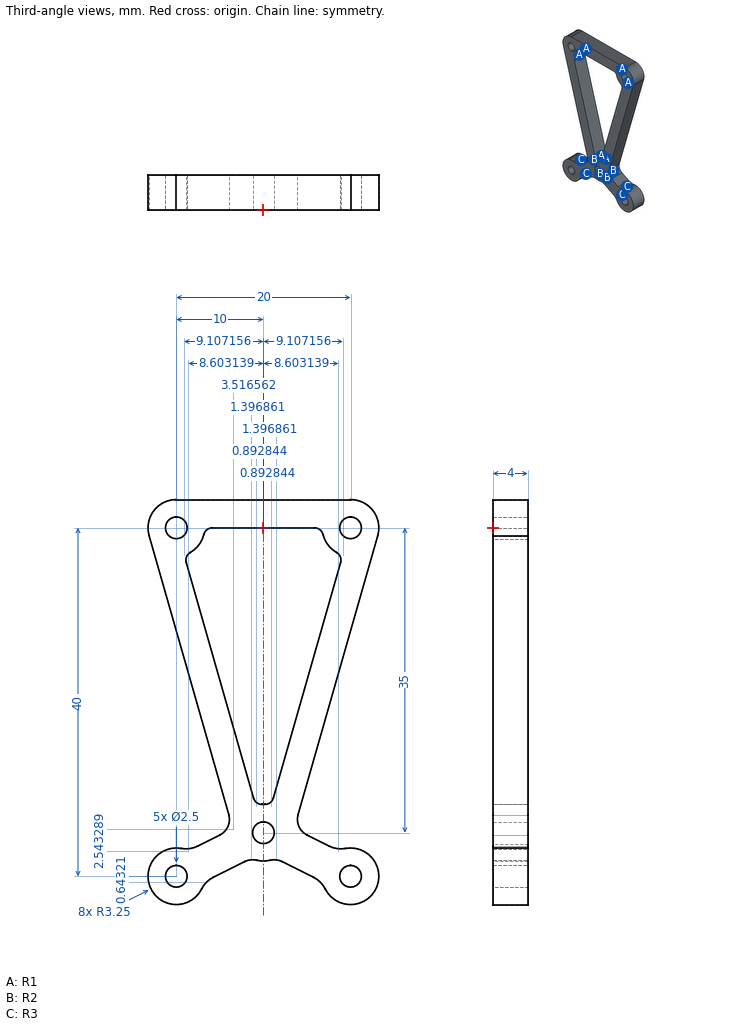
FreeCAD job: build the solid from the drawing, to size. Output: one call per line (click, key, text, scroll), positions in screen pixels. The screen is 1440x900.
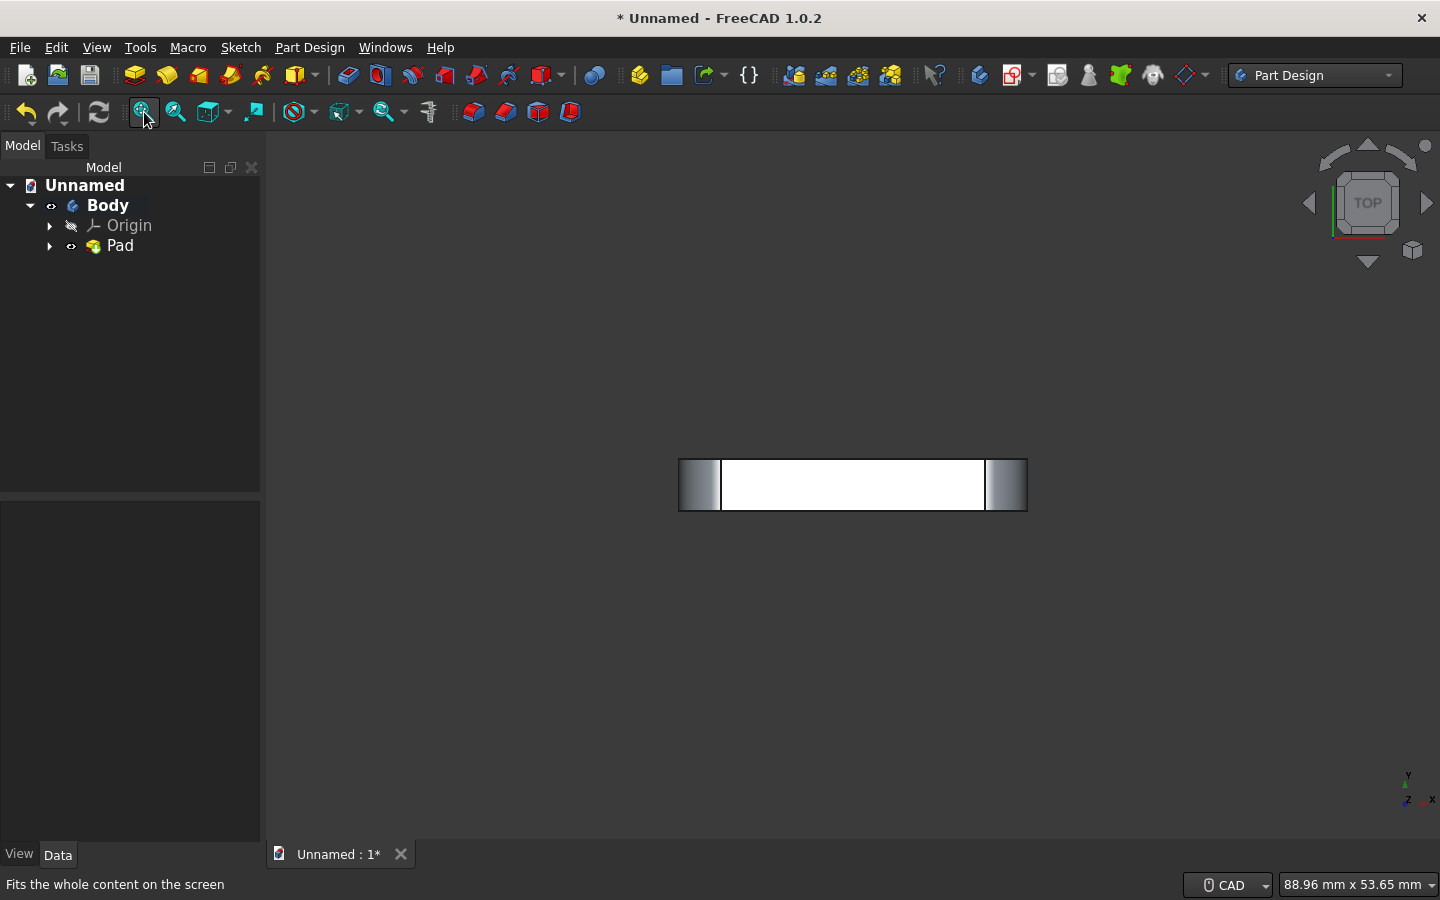
key(1)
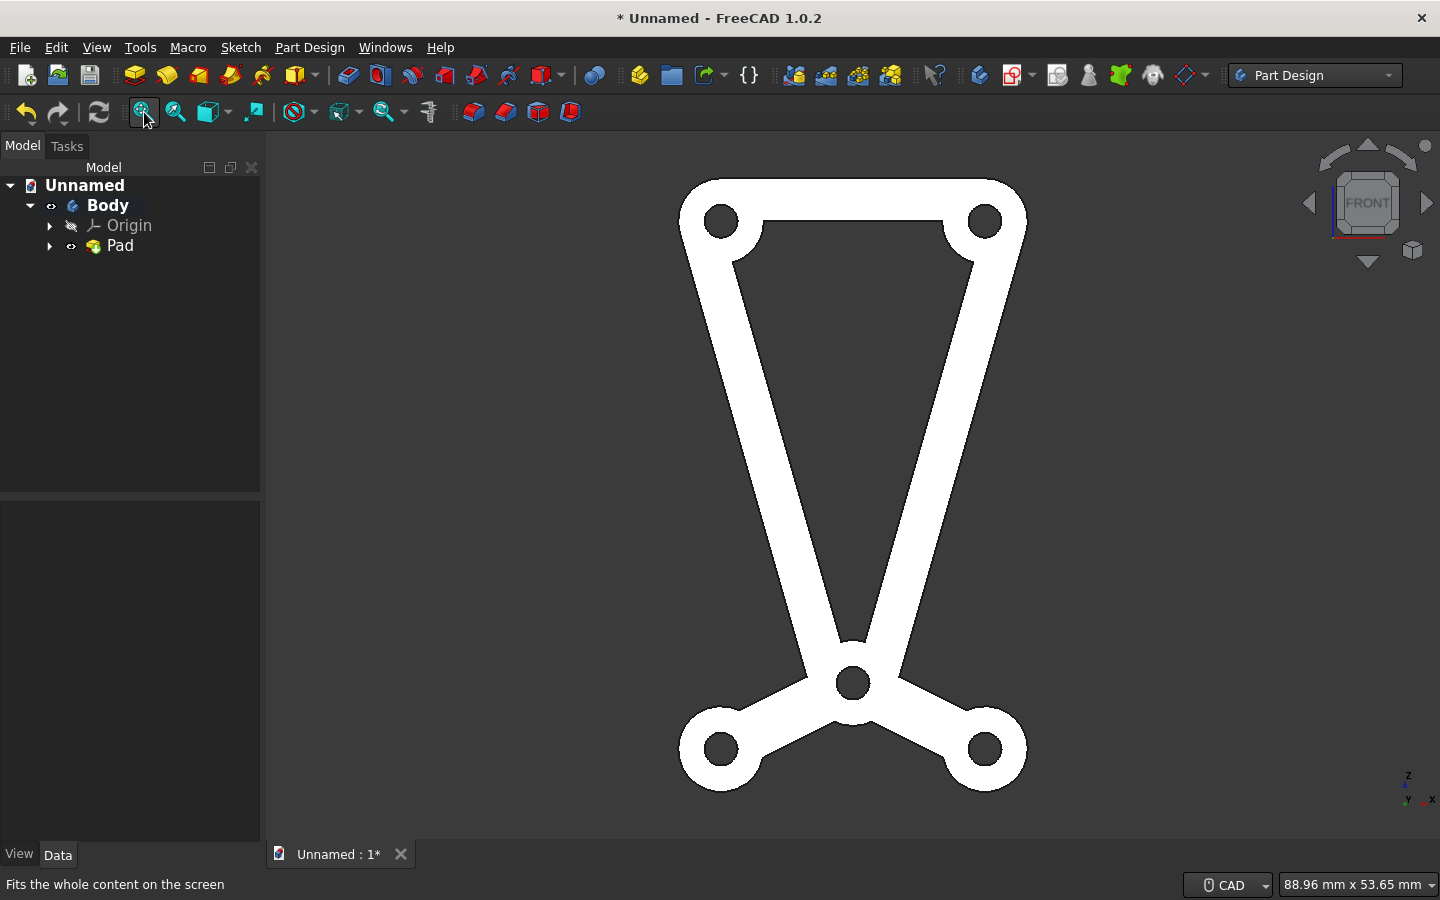
key(3)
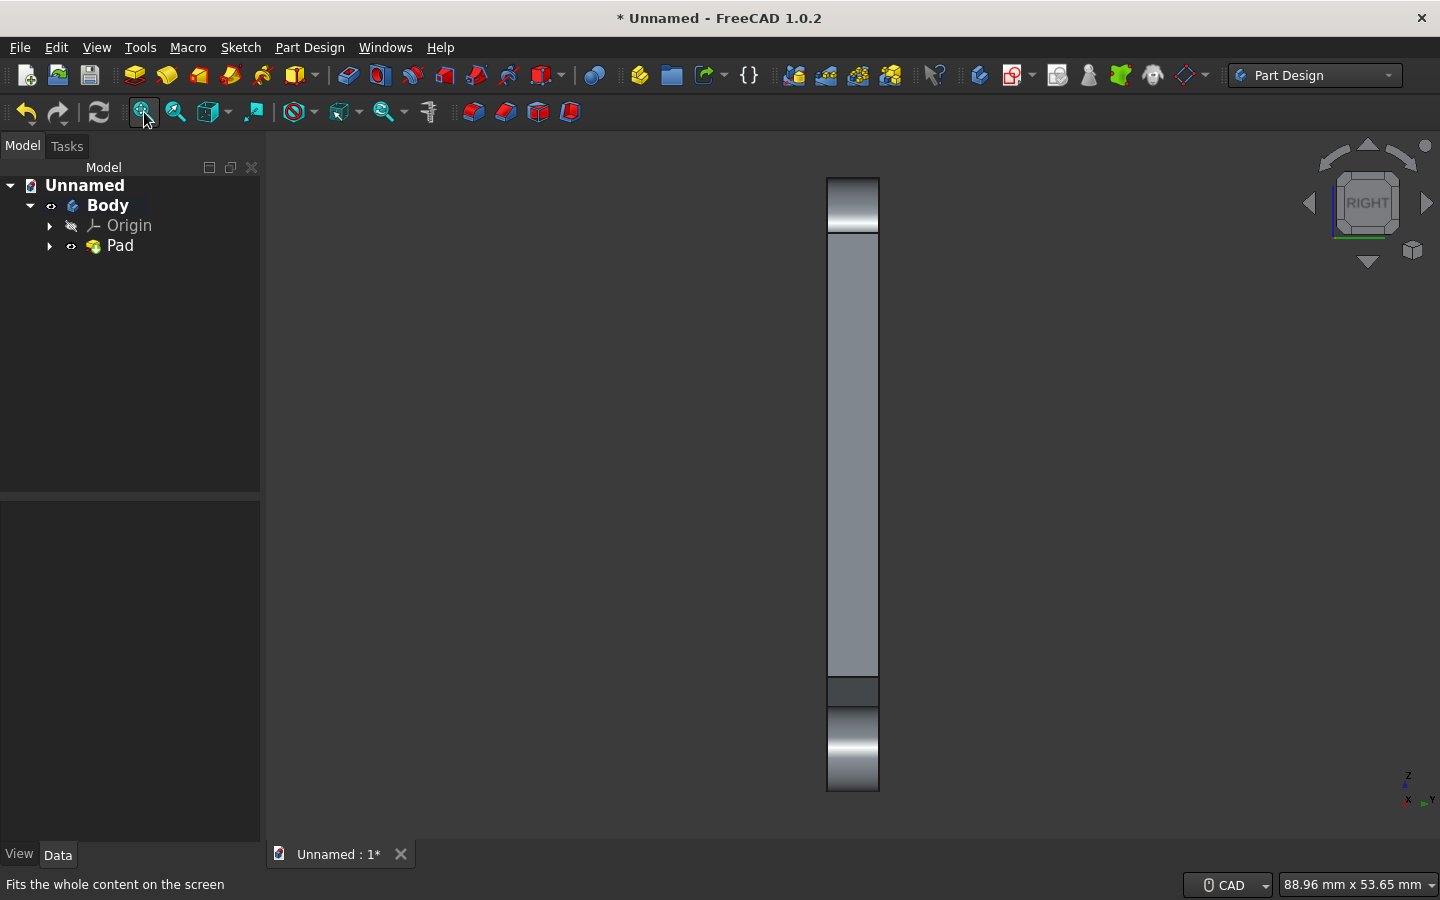
key(5)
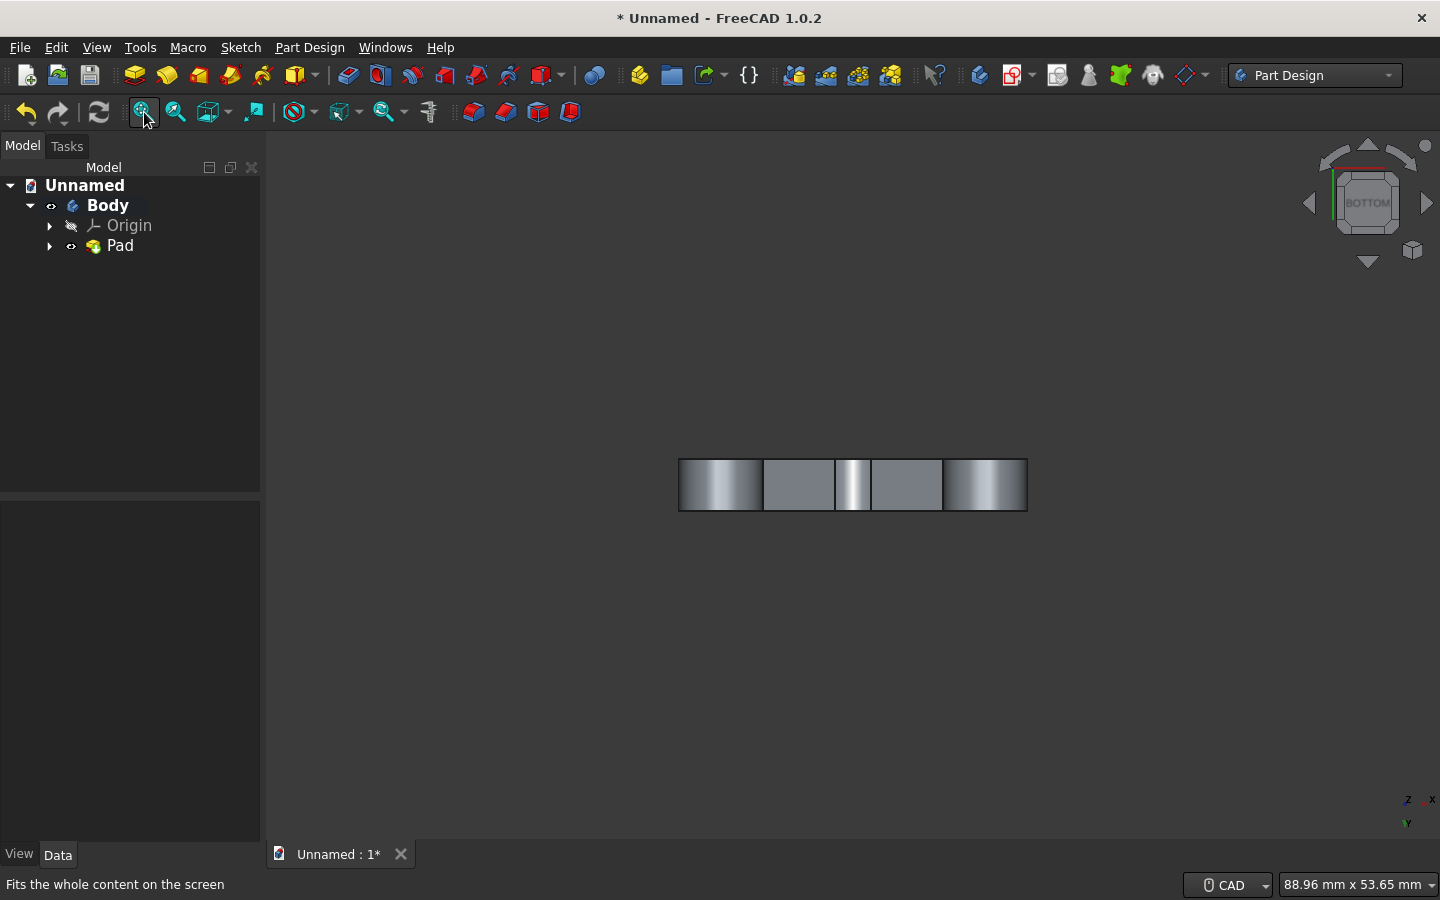
click(144, 112)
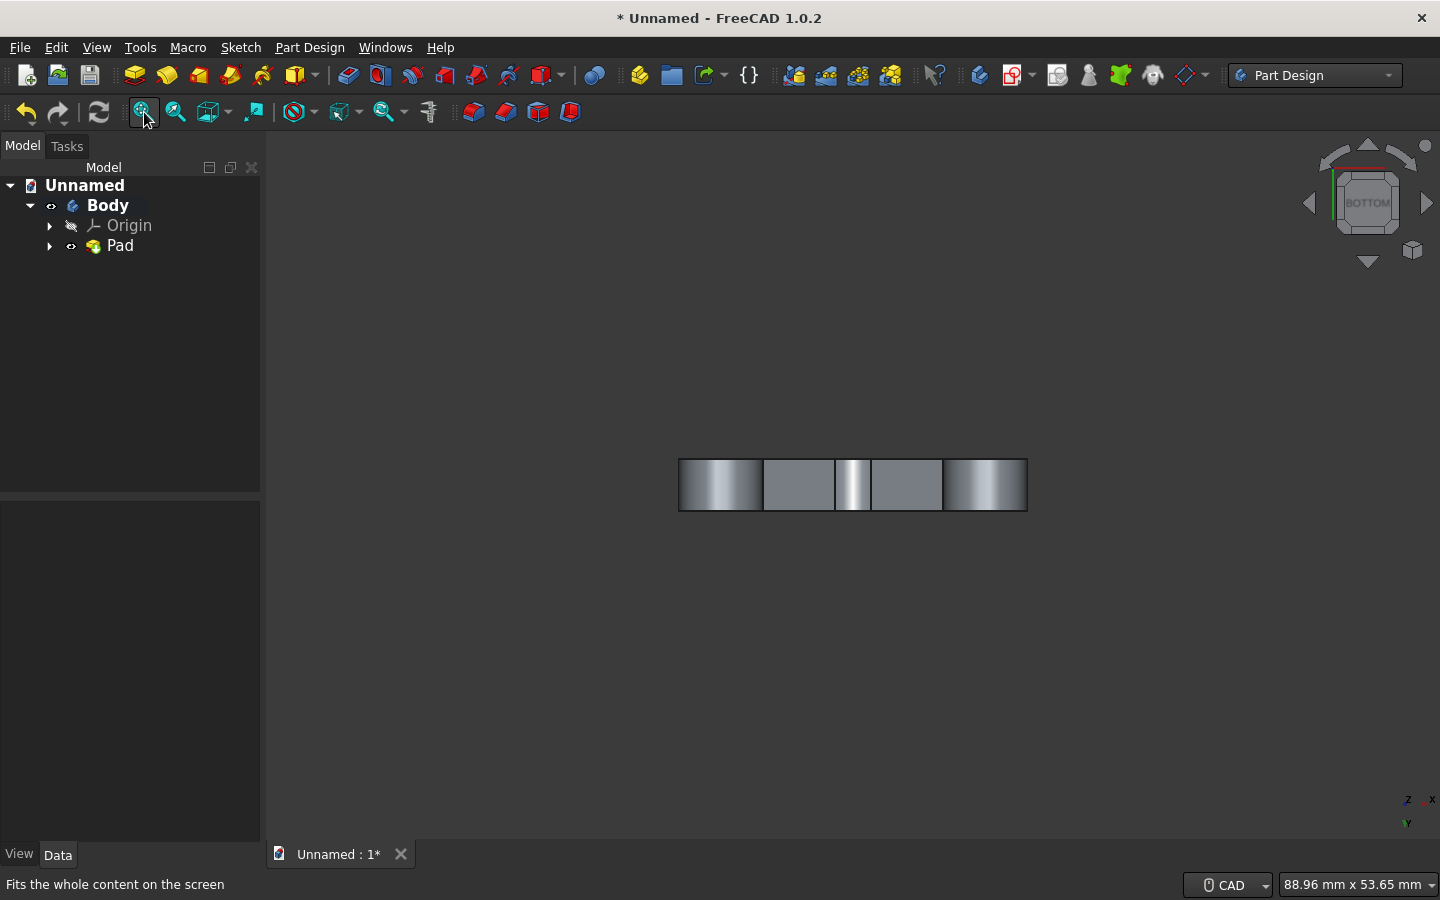
key(4)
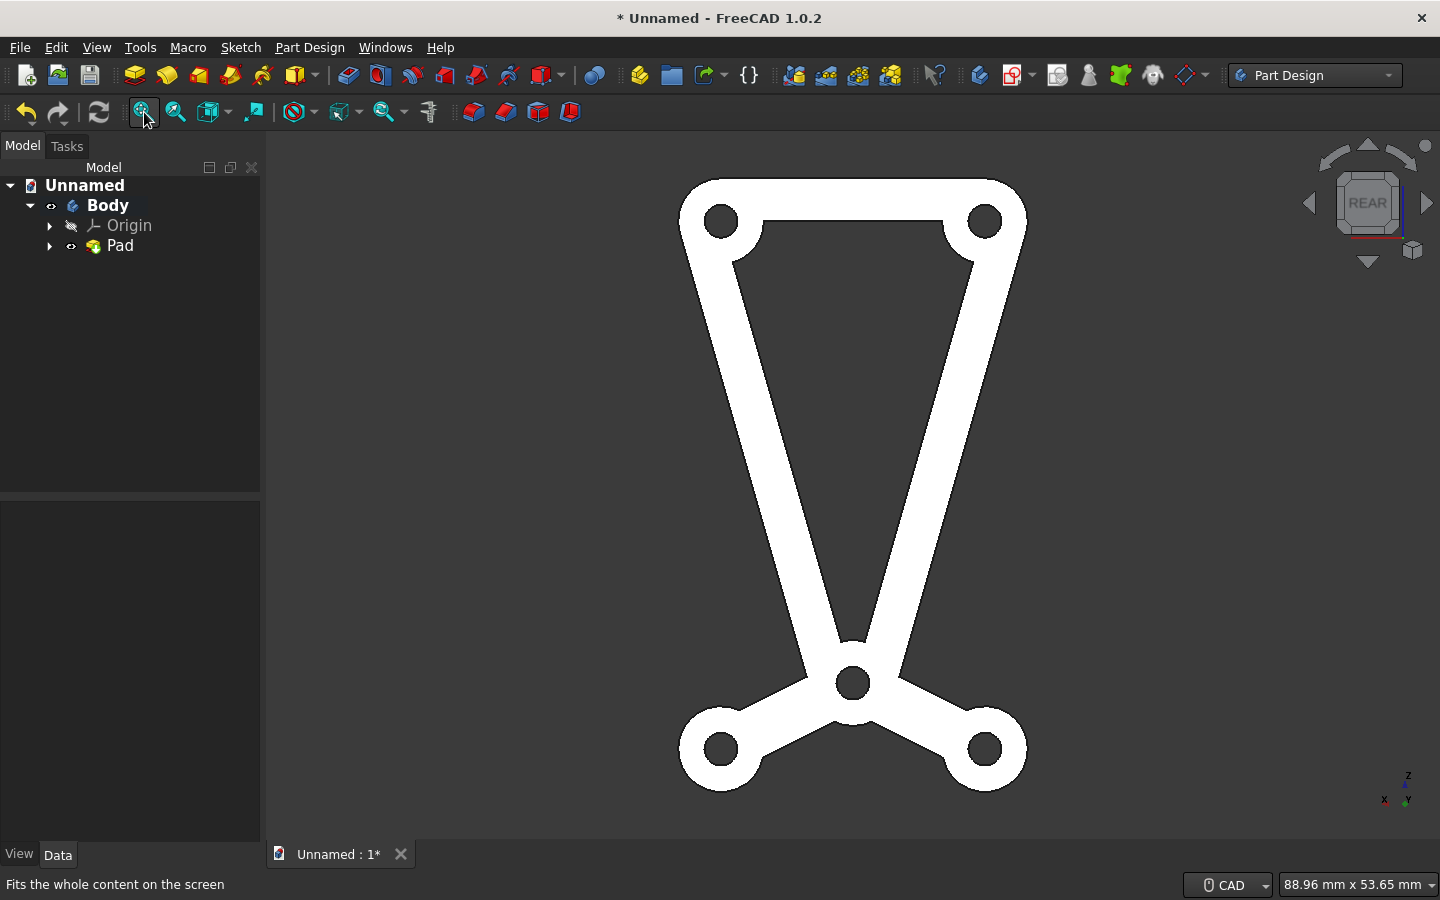
key(6)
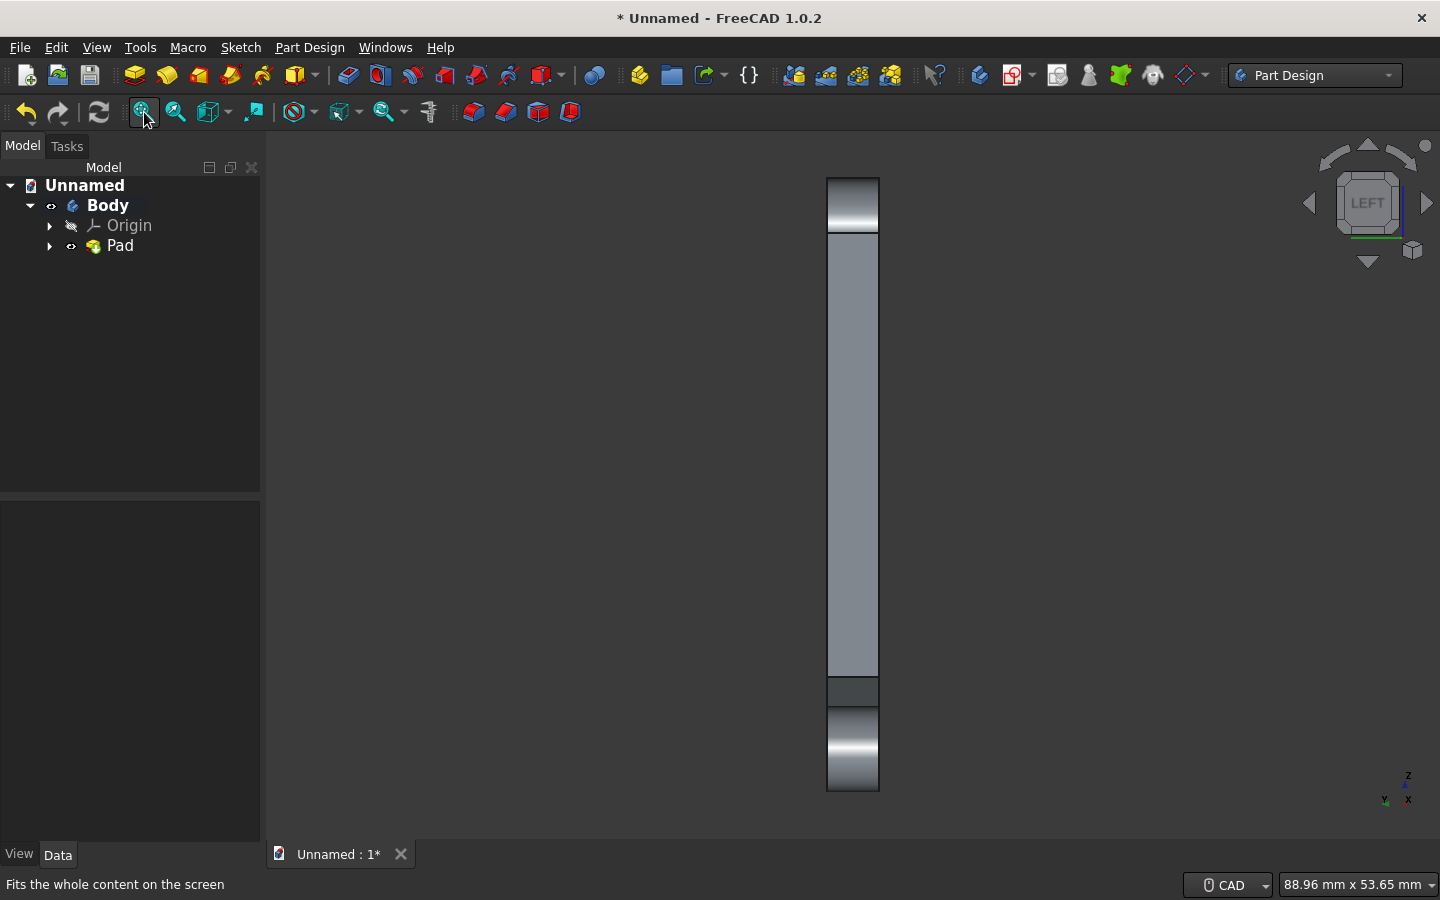
key(v)
key(3)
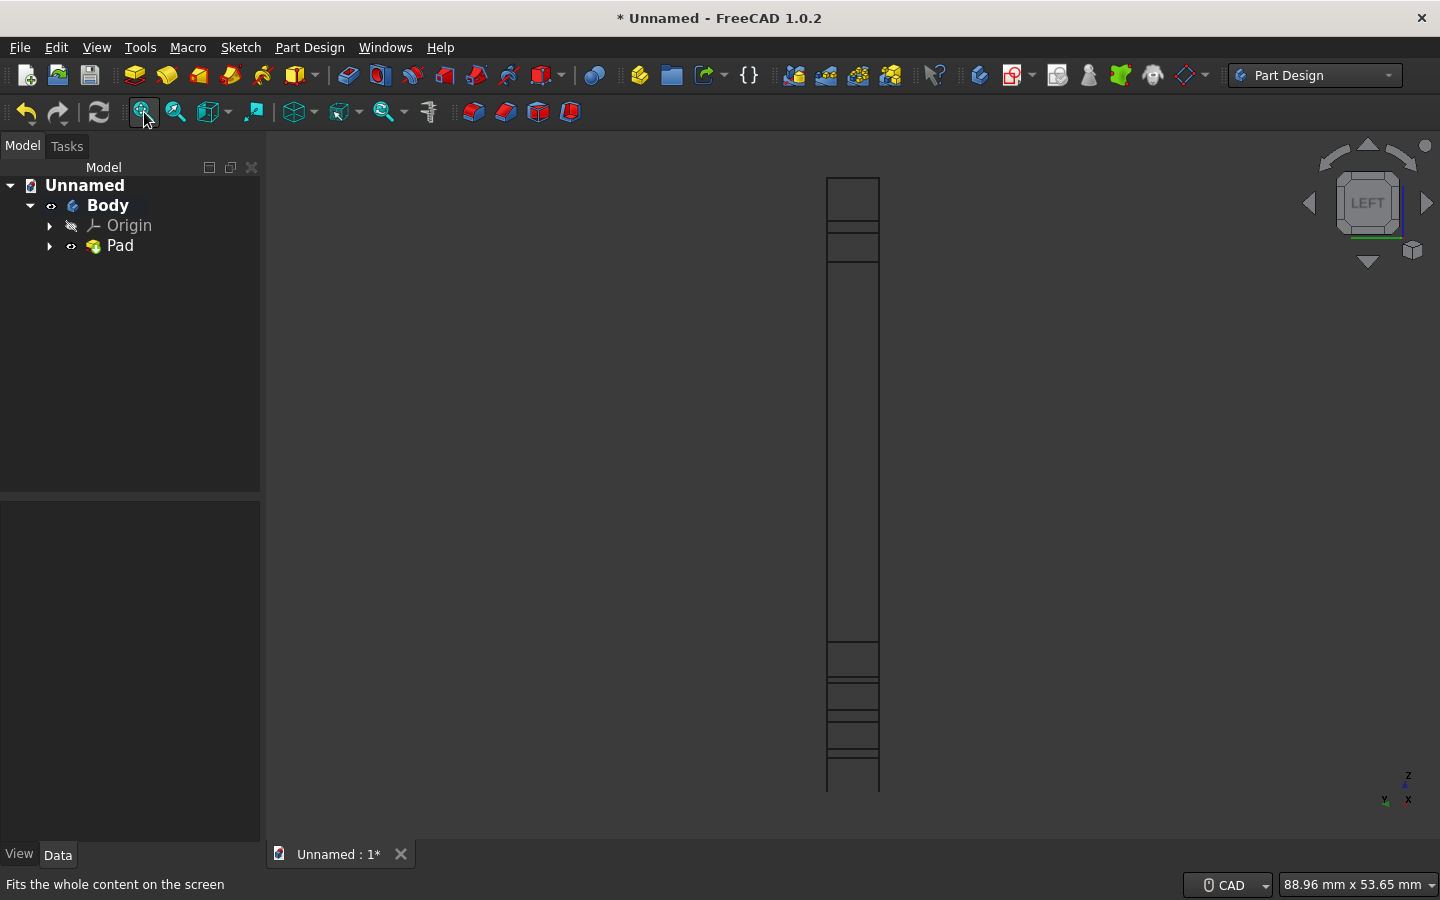
key(0)